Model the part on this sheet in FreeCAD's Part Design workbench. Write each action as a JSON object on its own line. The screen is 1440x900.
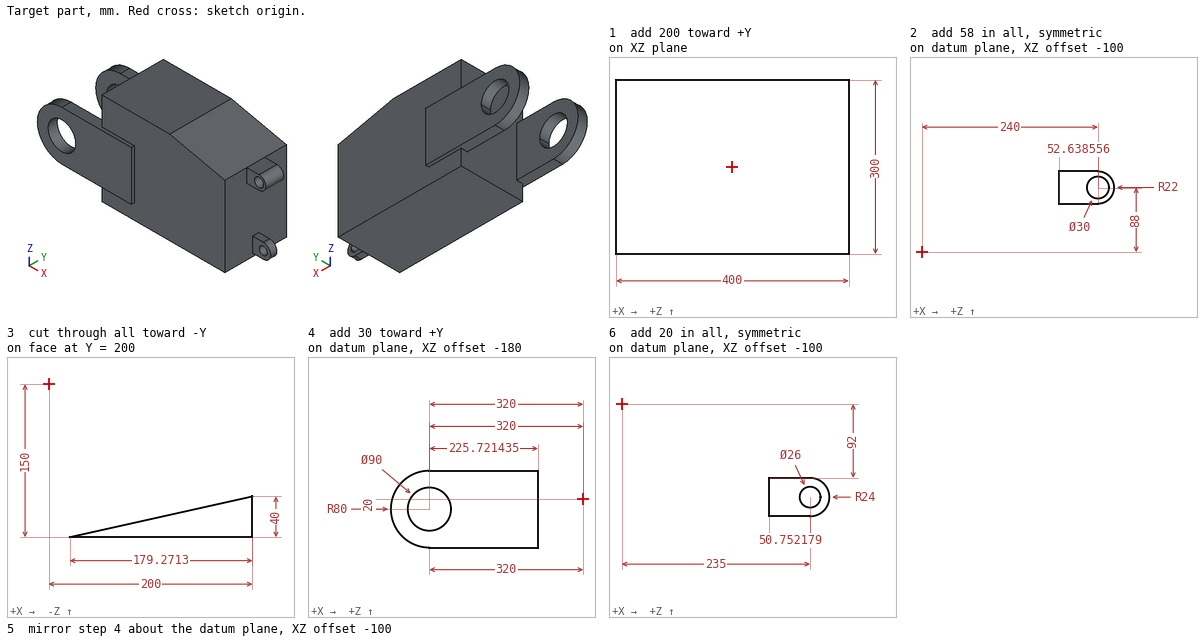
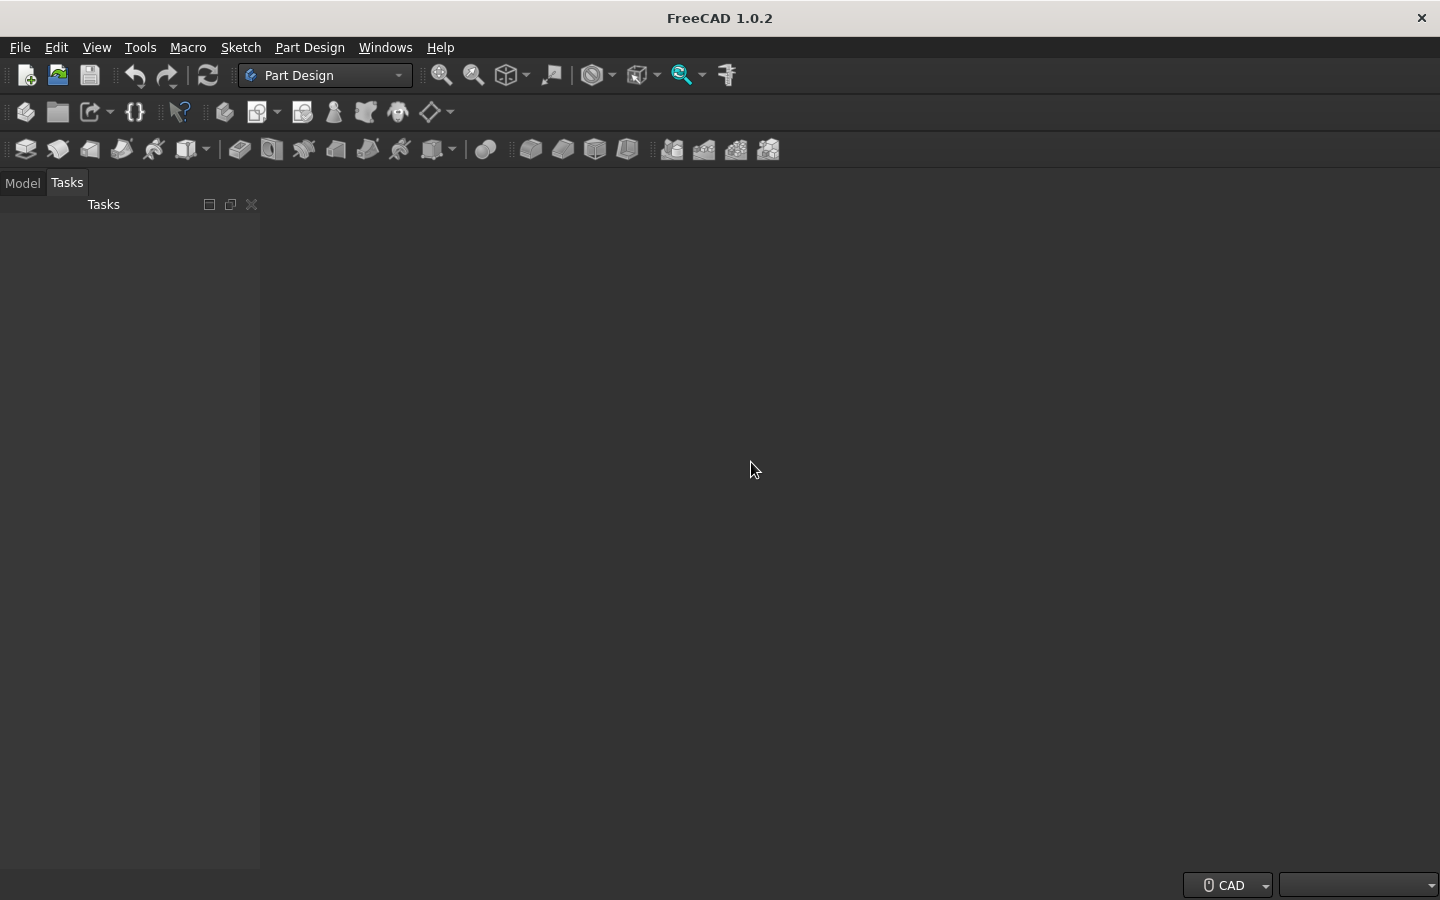
{"action": "left_click", "coordinate": [26, 76]}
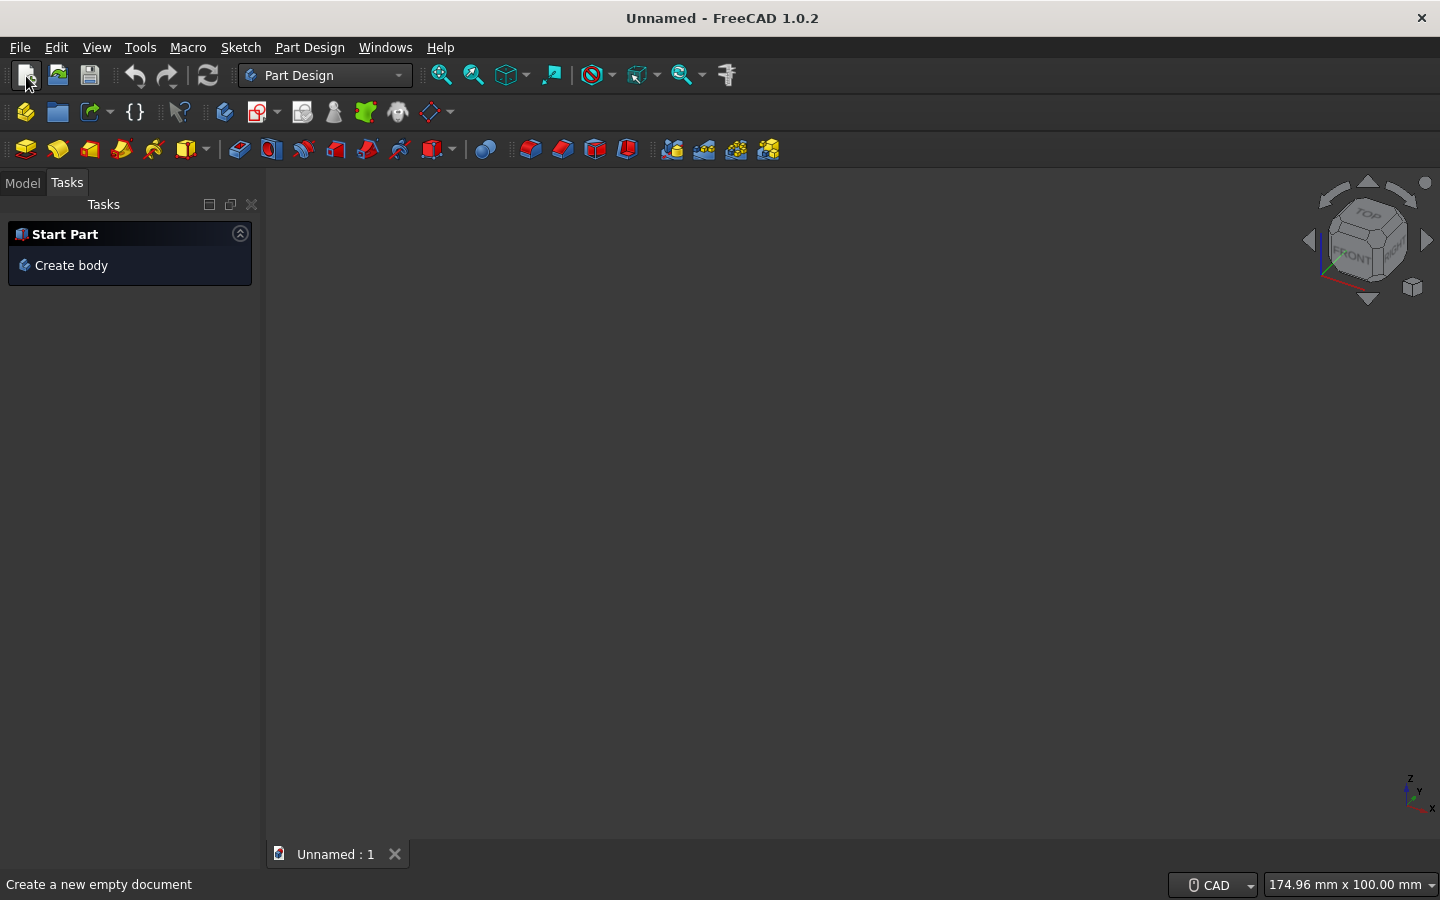
{"action": "left_click", "coordinate": [258, 112]}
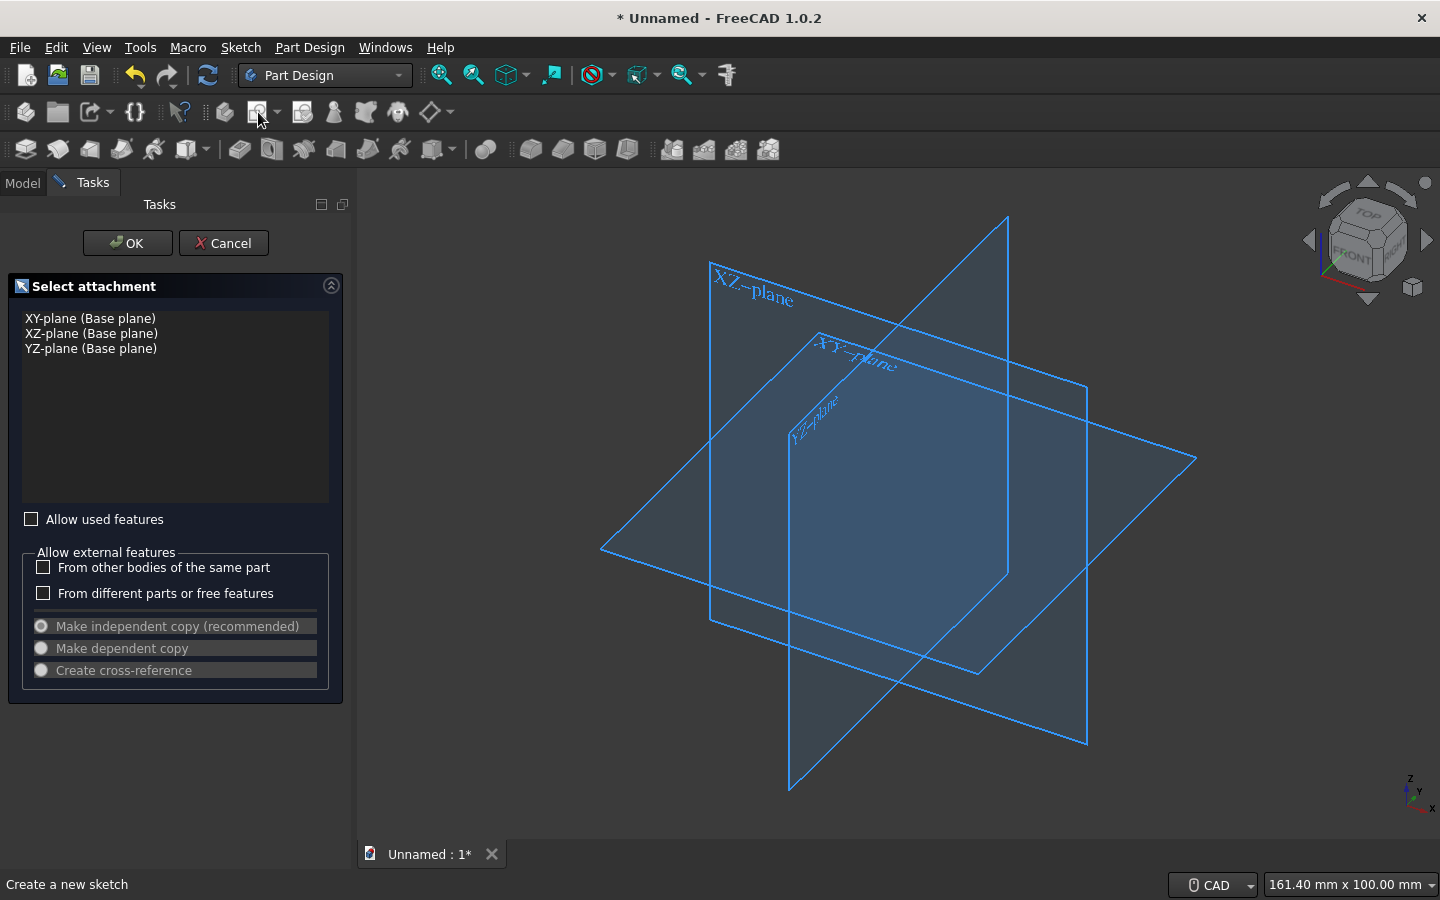
{"action": "left_click", "coordinate": [82, 334]}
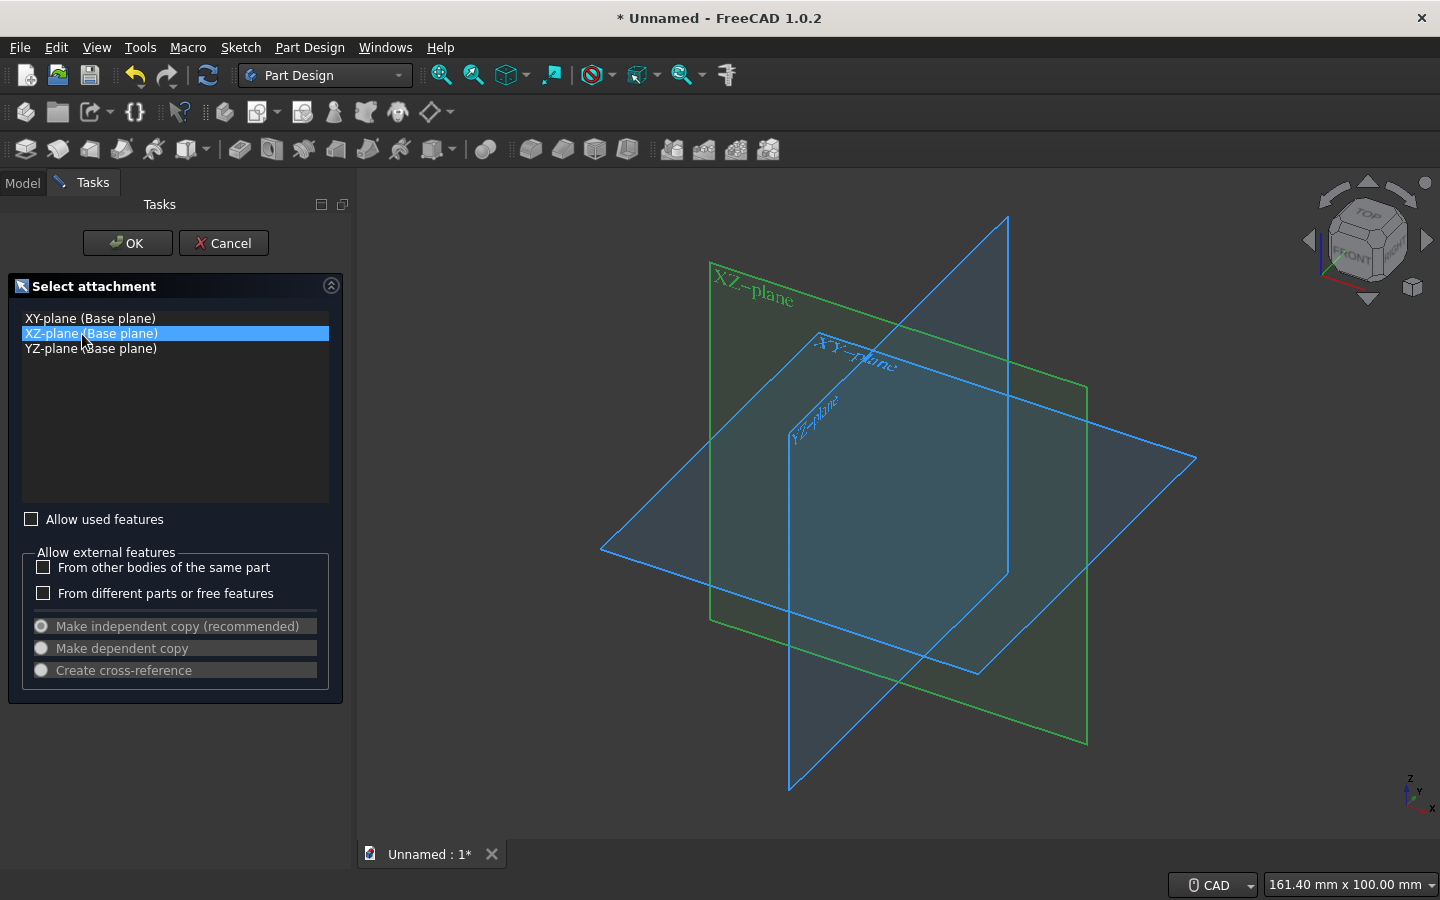
{"action": "left_click", "coordinate": [128, 243]}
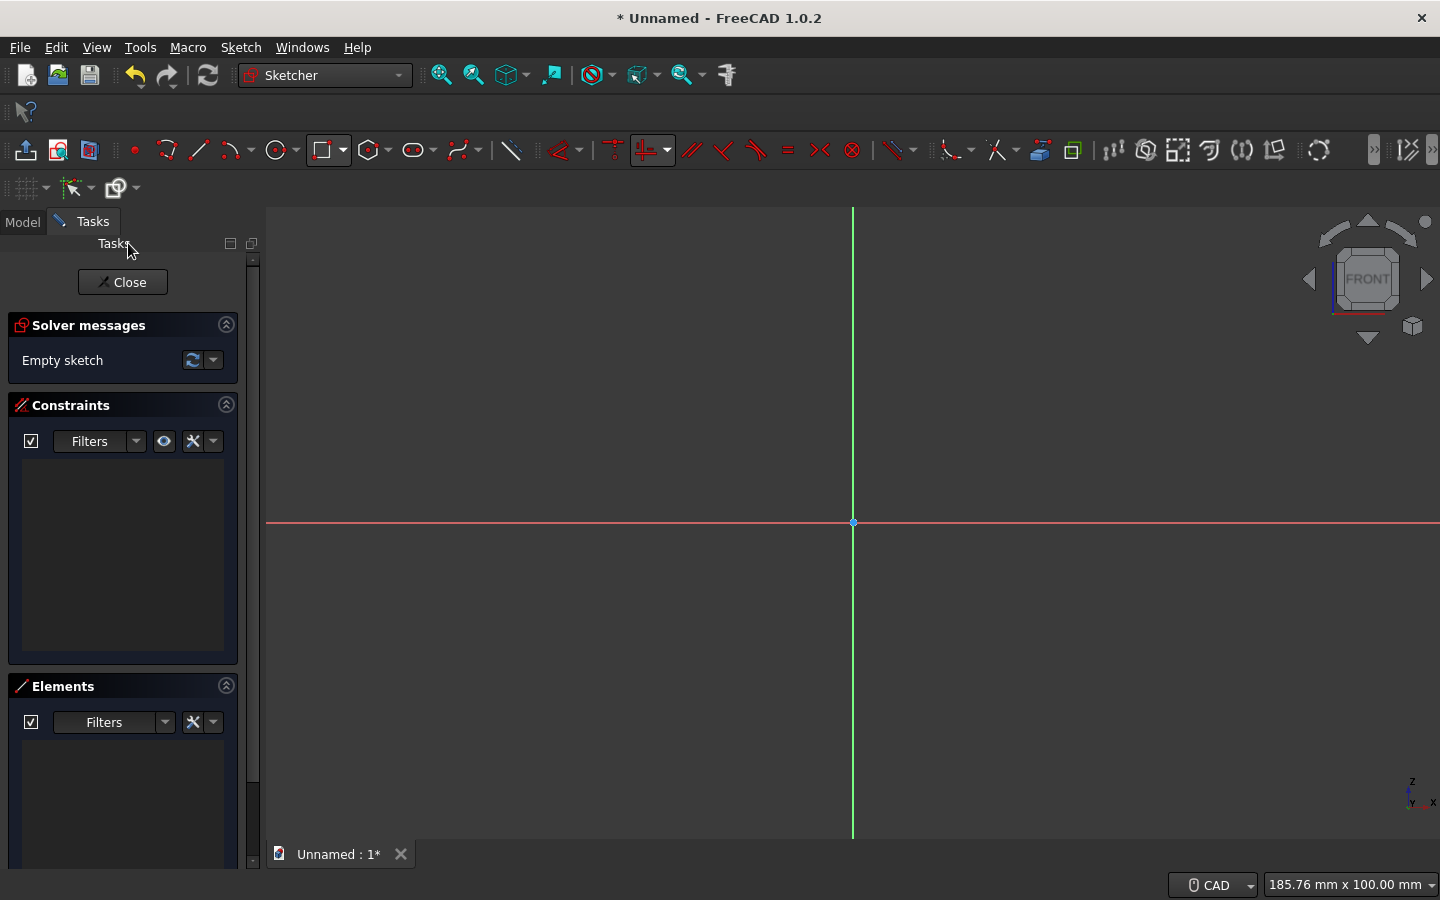
{"action": "scroll", "coordinate": [767, 523], "scroll_direction": "down", "scroll_amount": 8}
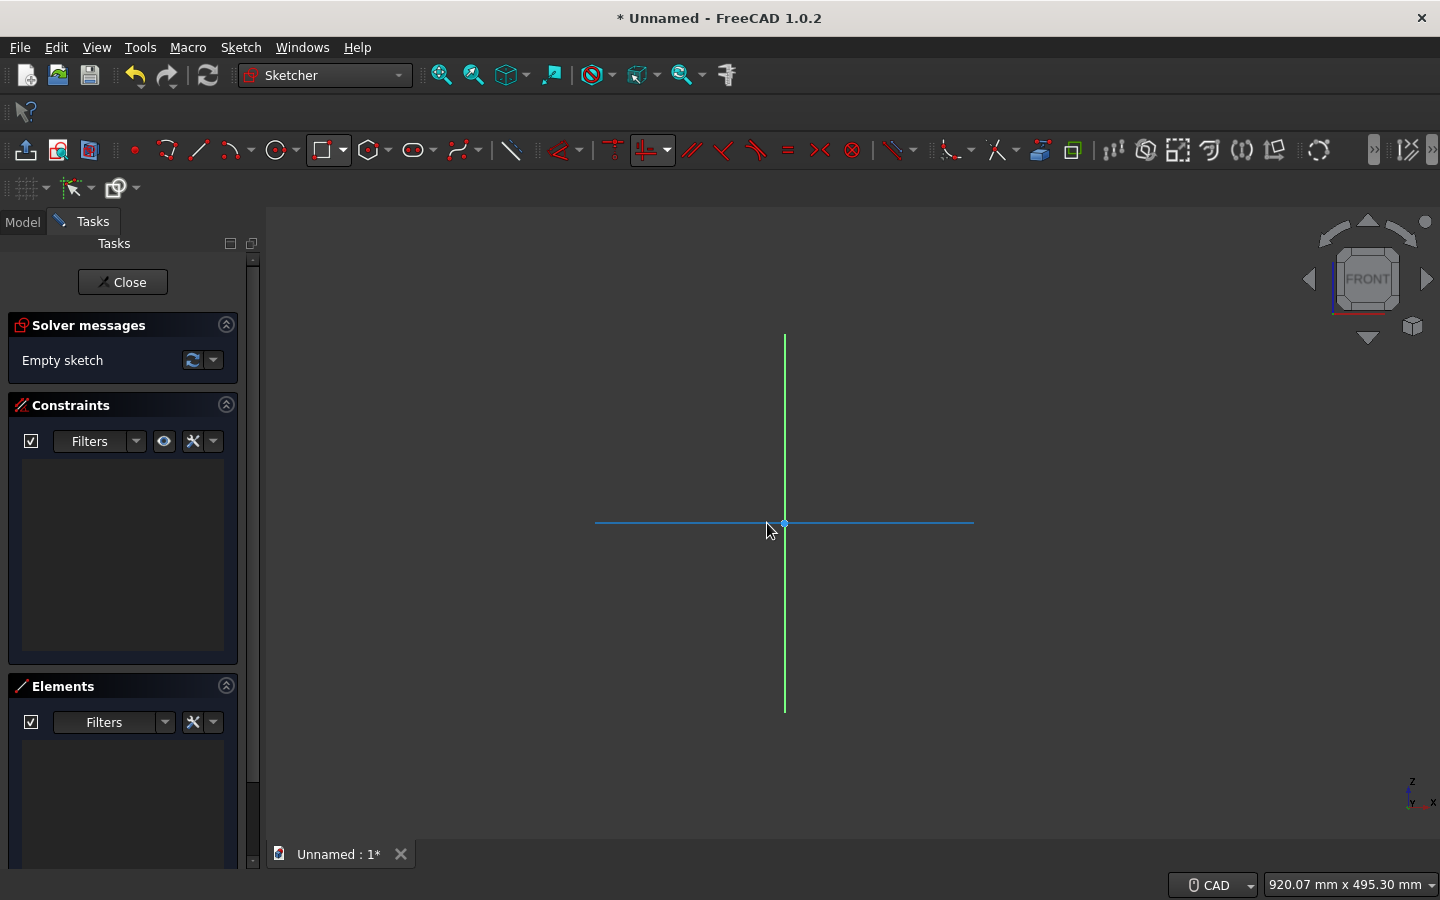
{"action": "left_click", "coordinate": [346, 150]}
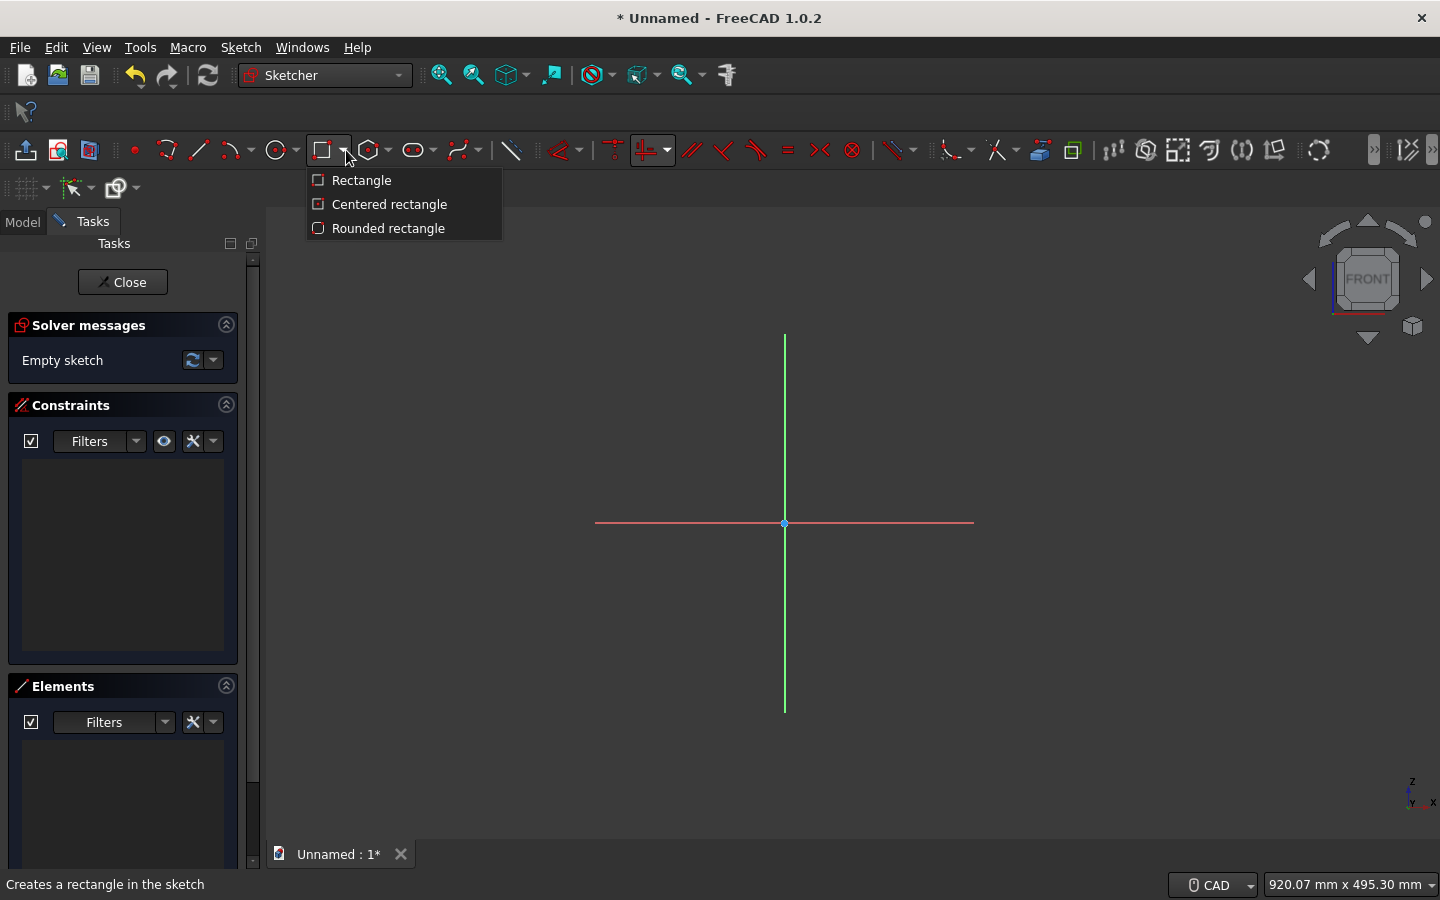
{"action": "left_click", "coordinate": [404, 204]}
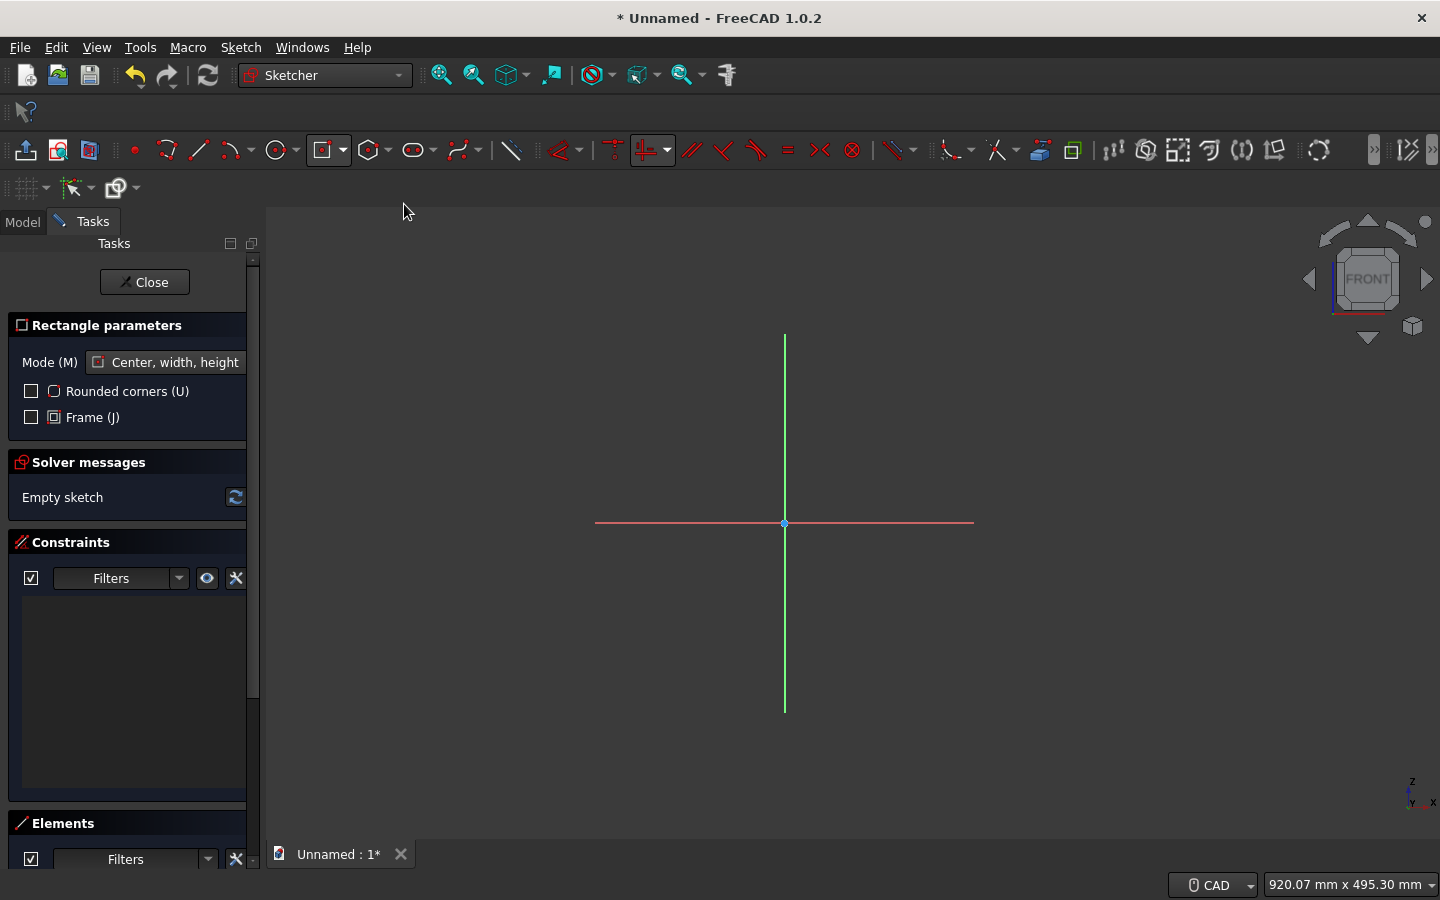
{"action": "left_click", "coordinate": [785, 523]}
{"action": "left_click", "coordinate": [1040, 332]}
{"action": "key", "text": "Escape"}